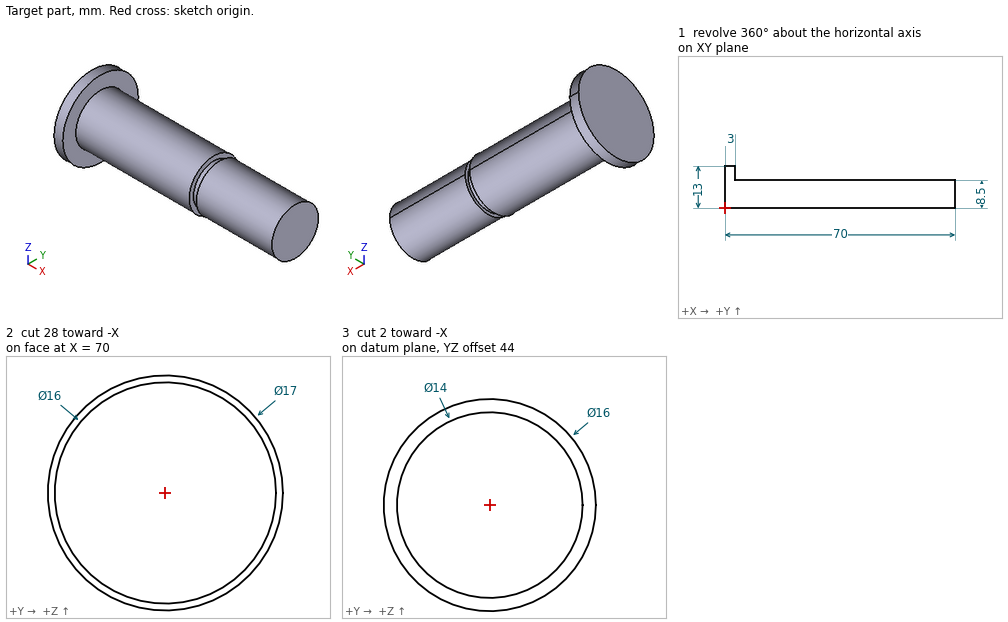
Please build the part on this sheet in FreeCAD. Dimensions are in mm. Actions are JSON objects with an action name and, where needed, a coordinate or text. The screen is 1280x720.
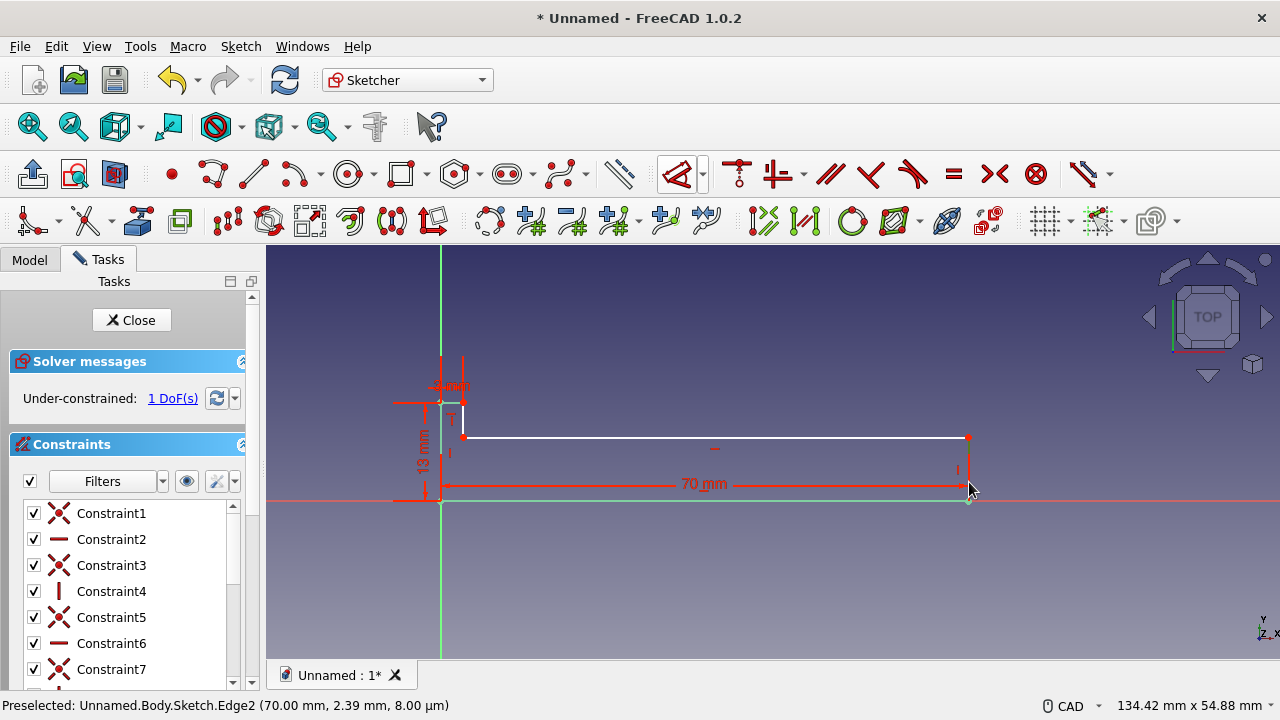
{"action": "key", "text": "i"}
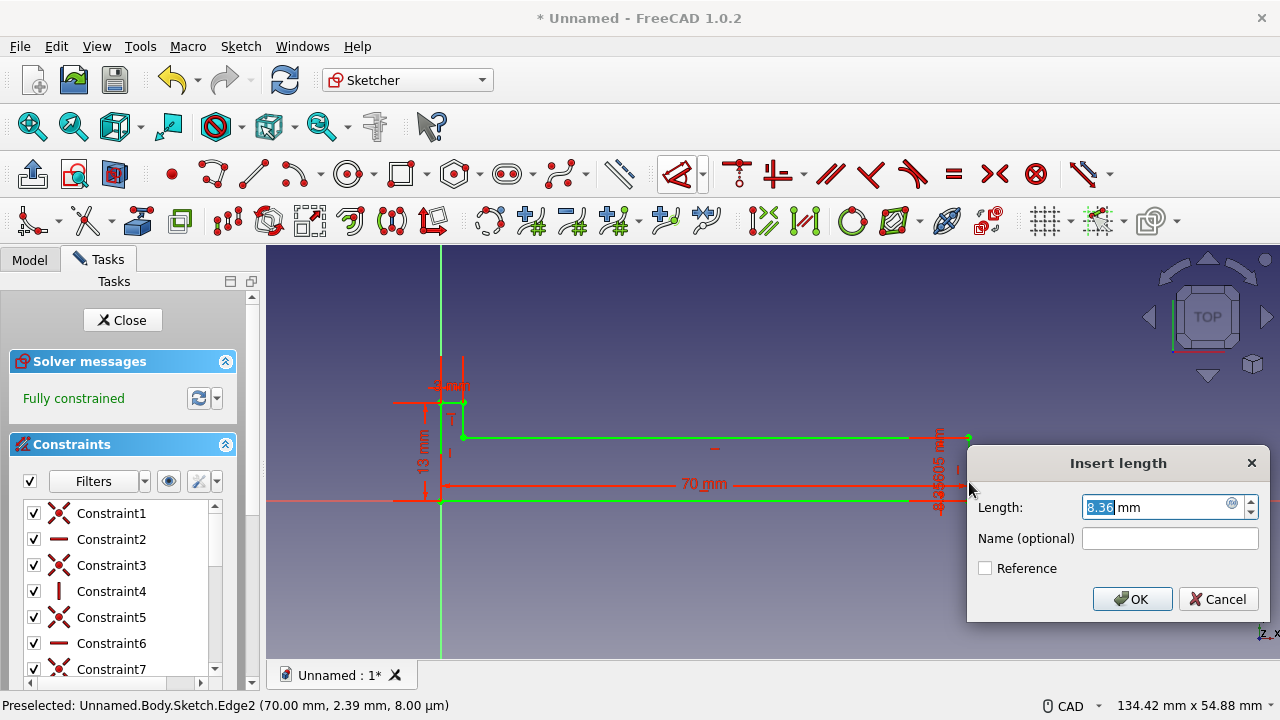
{"action": "type", "text": "8.5"}
{"action": "key", "text": "Return"}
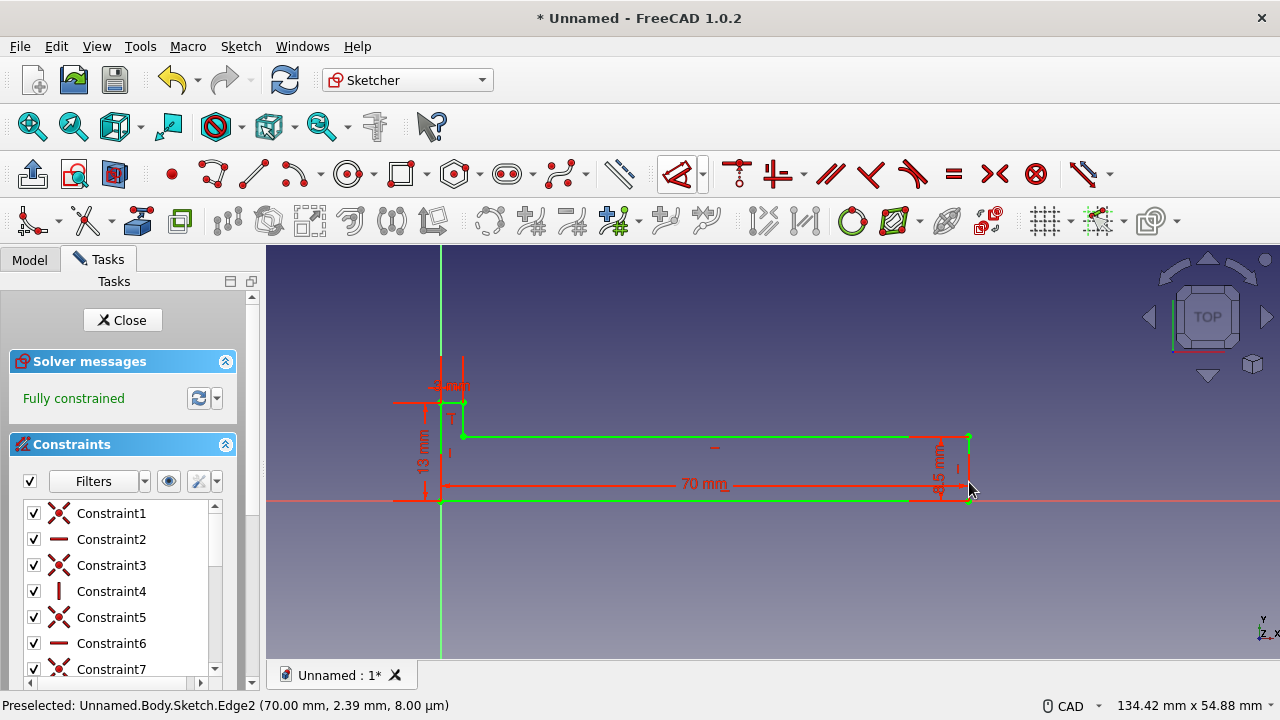
{"action": "left_click", "coordinate": [123, 320]}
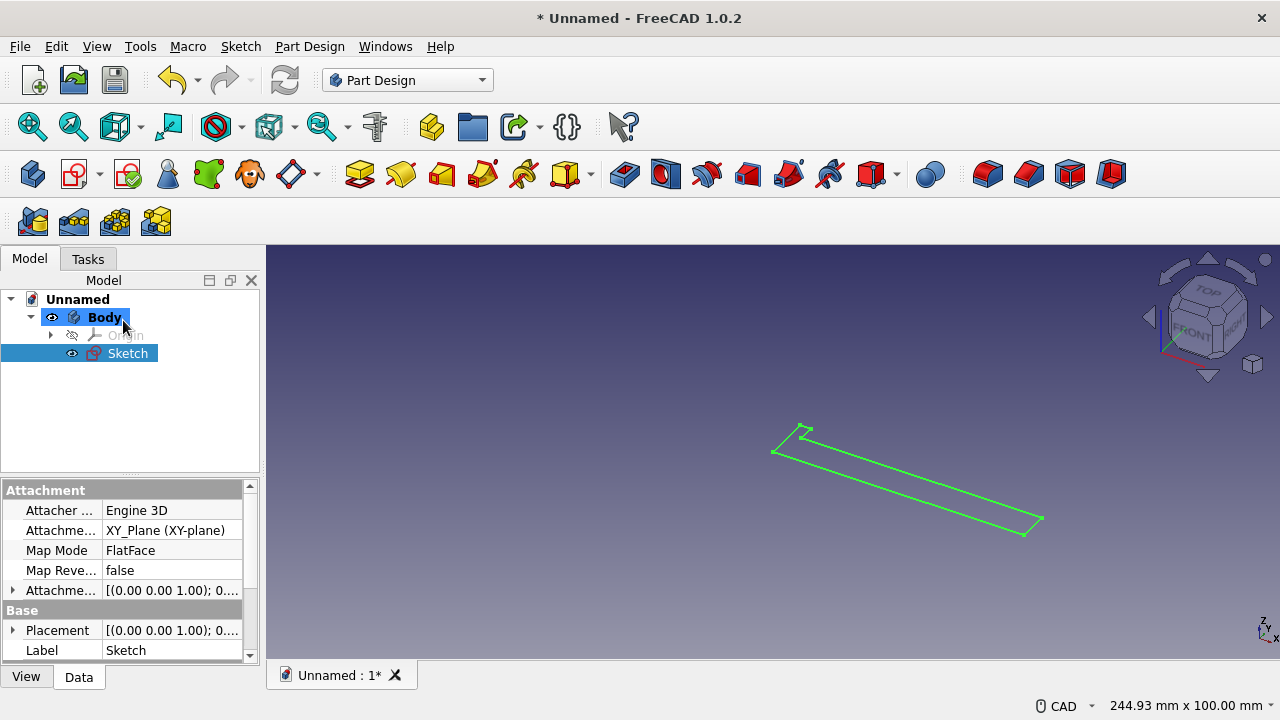
{"action": "left_click", "coordinate": [401, 174]}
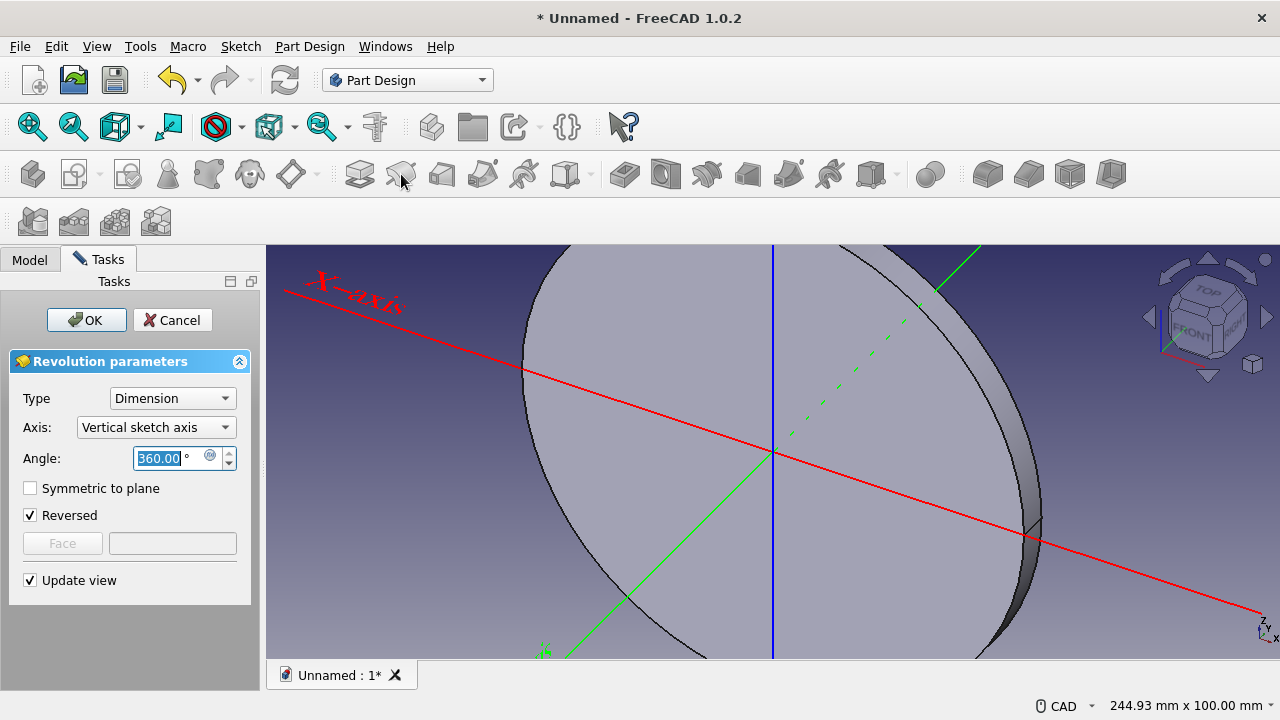
{"action": "left_click", "coordinate": [157, 428]}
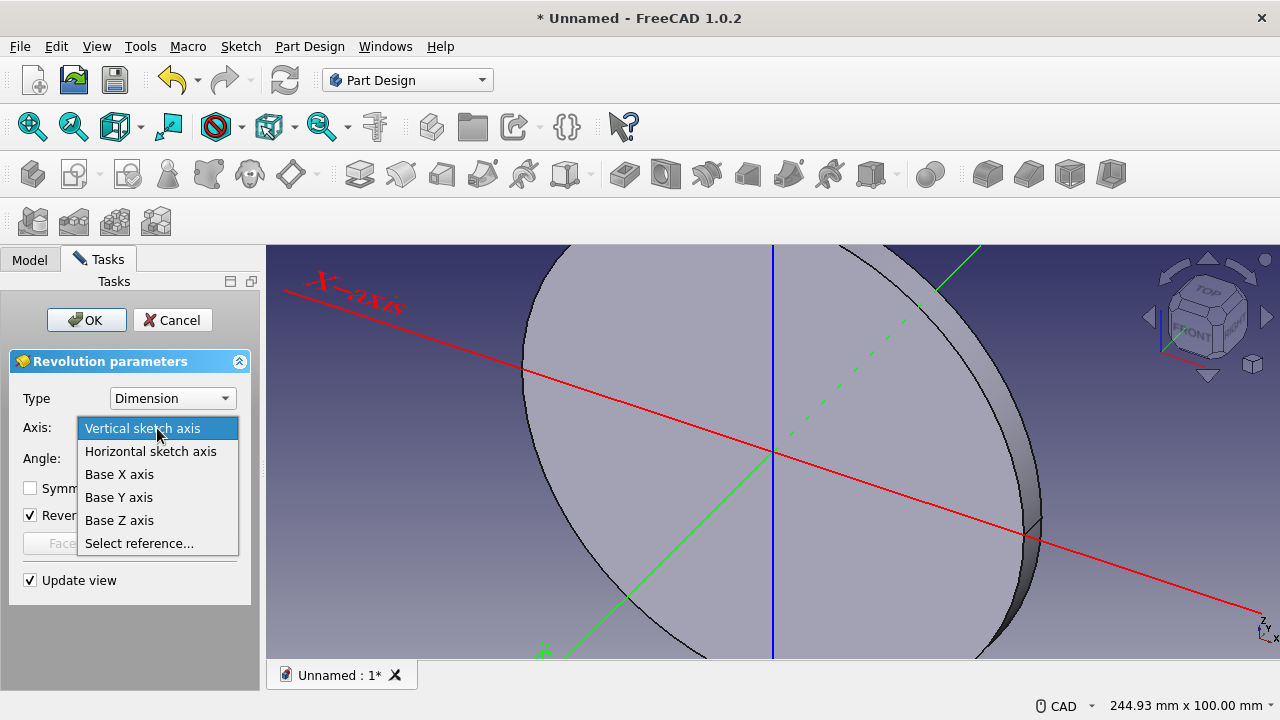
{"action": "left_click", "coordinate": [156, 452]}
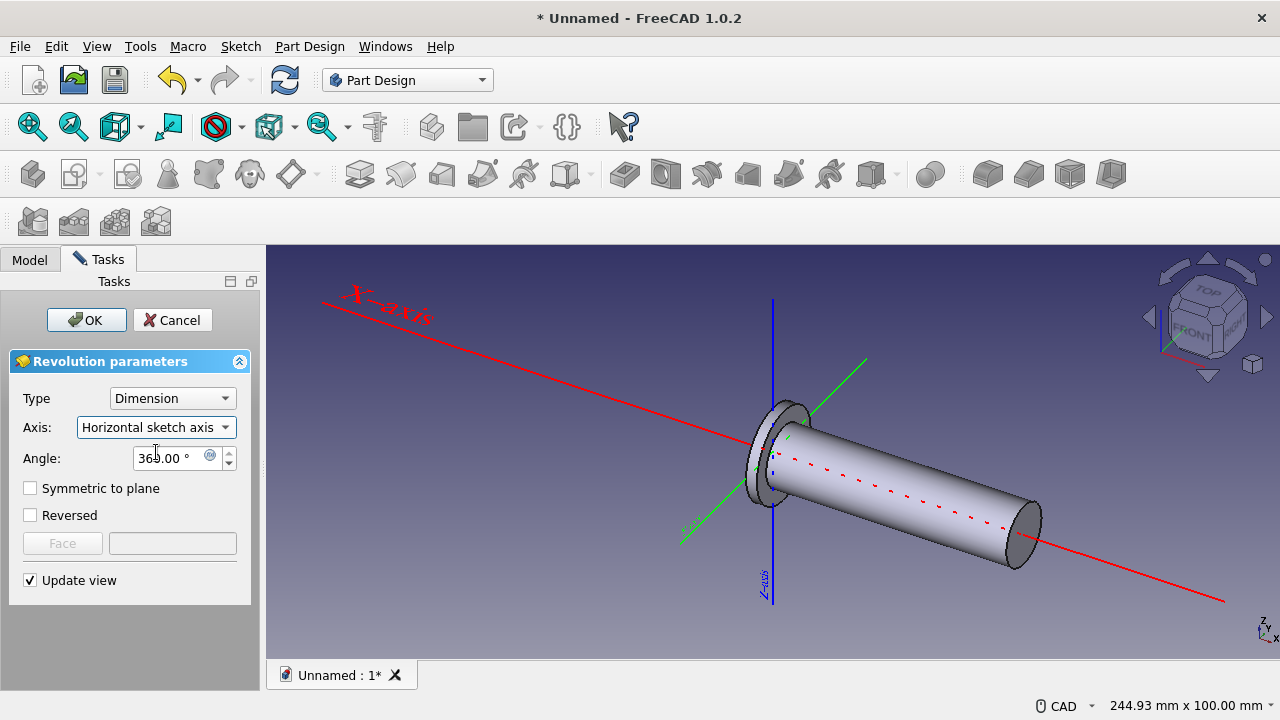
{"action": "left_click", "coordinate": [87, 320]}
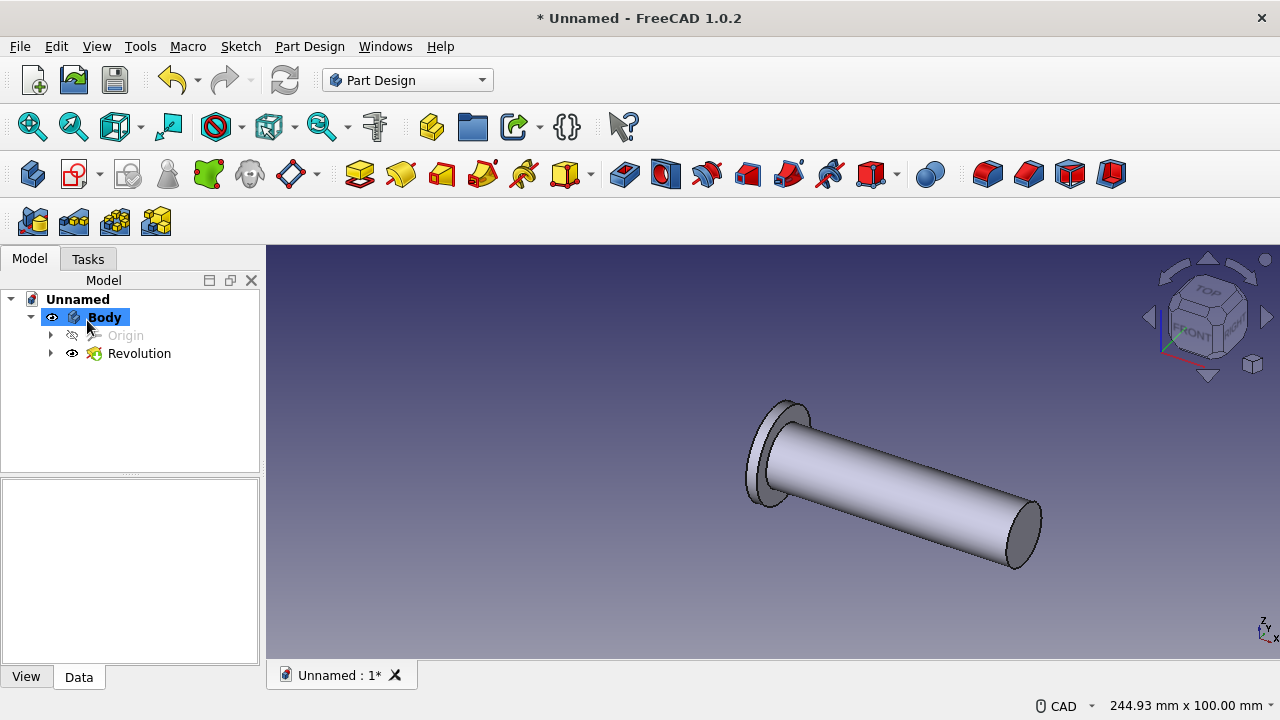
{"action": "left_click", "coordinate": [1024, 534]}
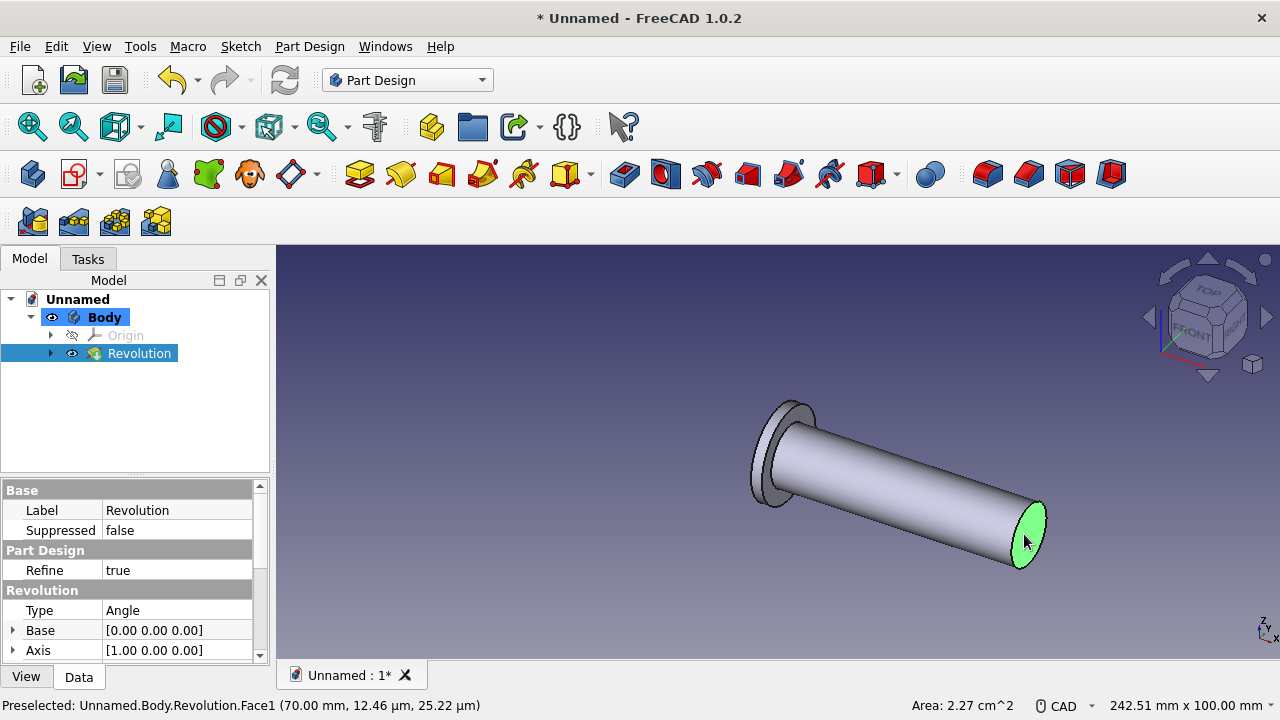
{"action": "left_click", "coordinate": [74, 174]}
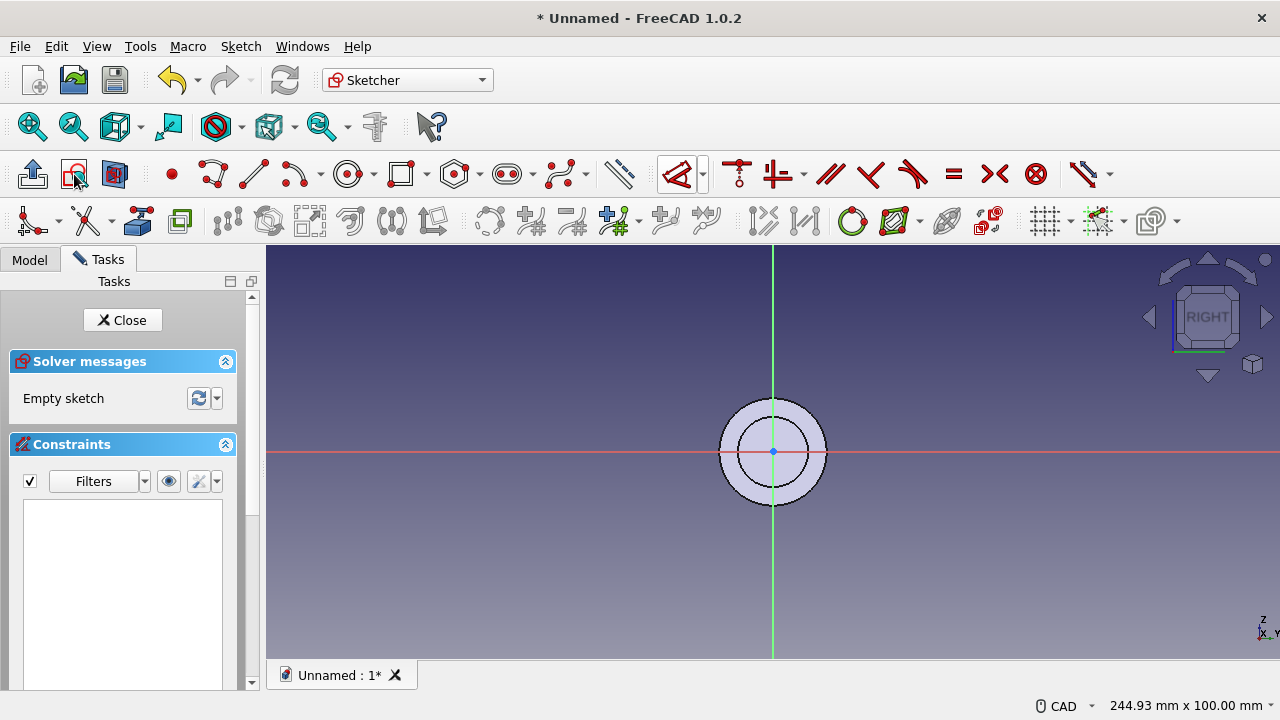
{"action": "scroll", "coordinate": [803, 452], "scroll_direction": "up", "scroll_amount": 6}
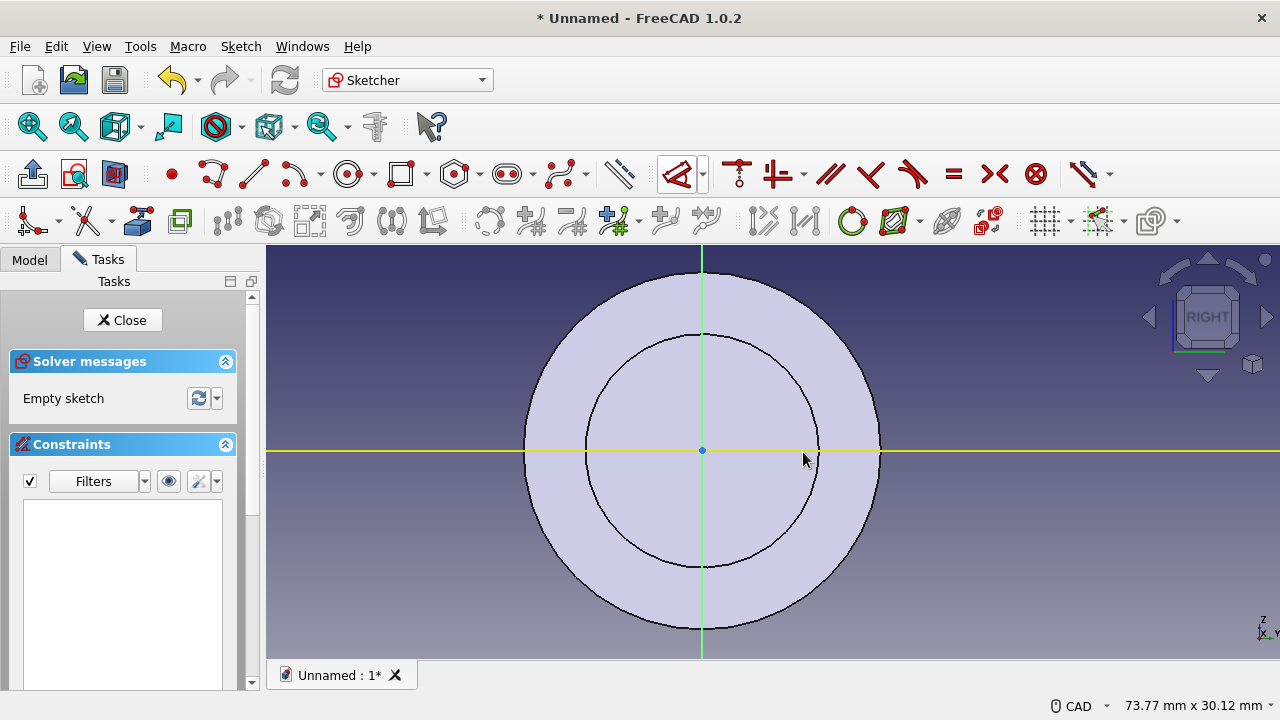
{"action": "key", "text": "g c"}